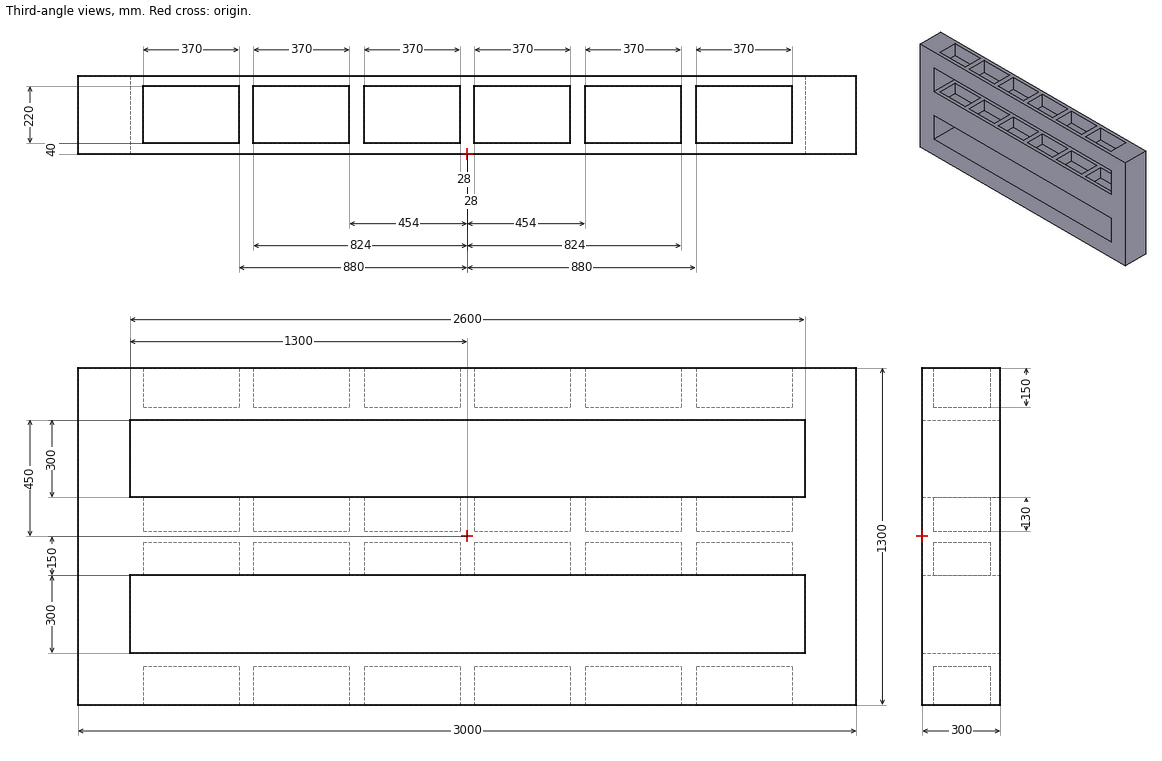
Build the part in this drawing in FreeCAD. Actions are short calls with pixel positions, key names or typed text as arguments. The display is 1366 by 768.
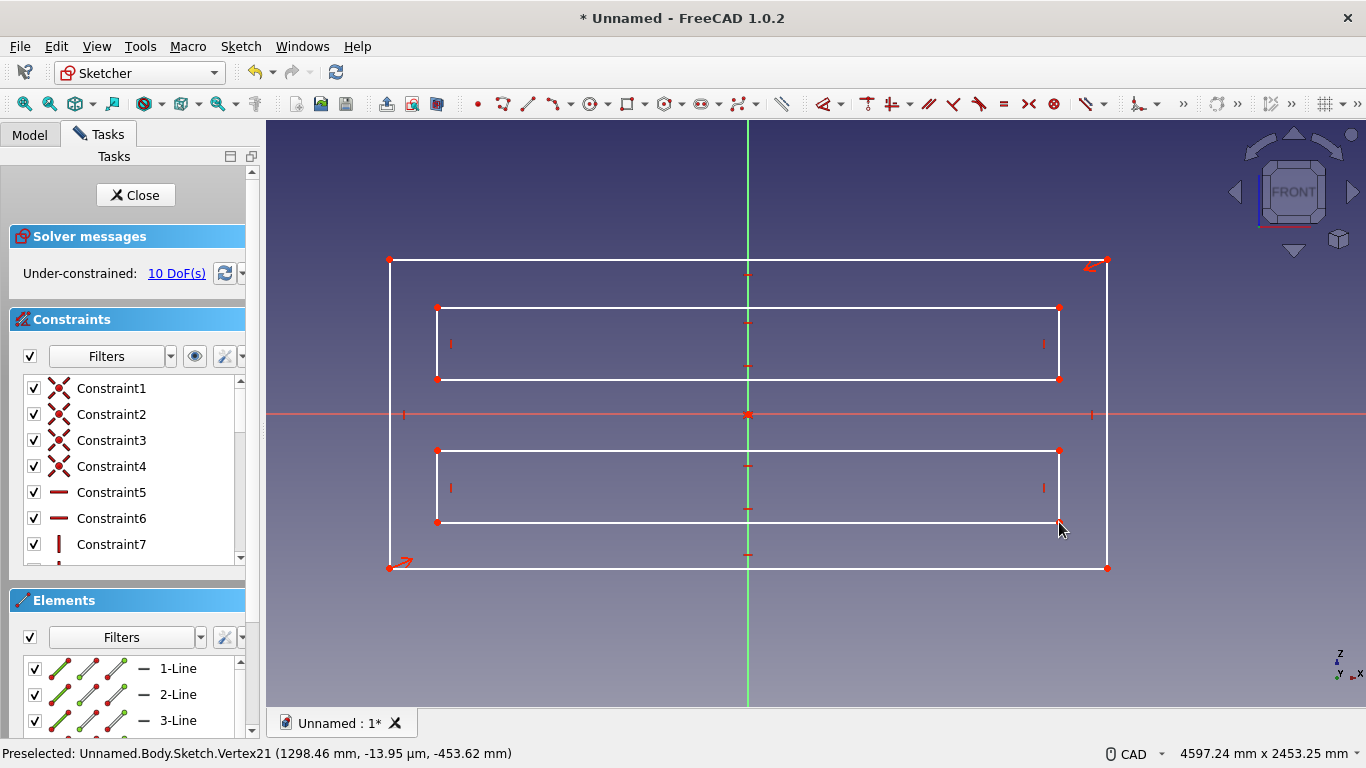
key(d)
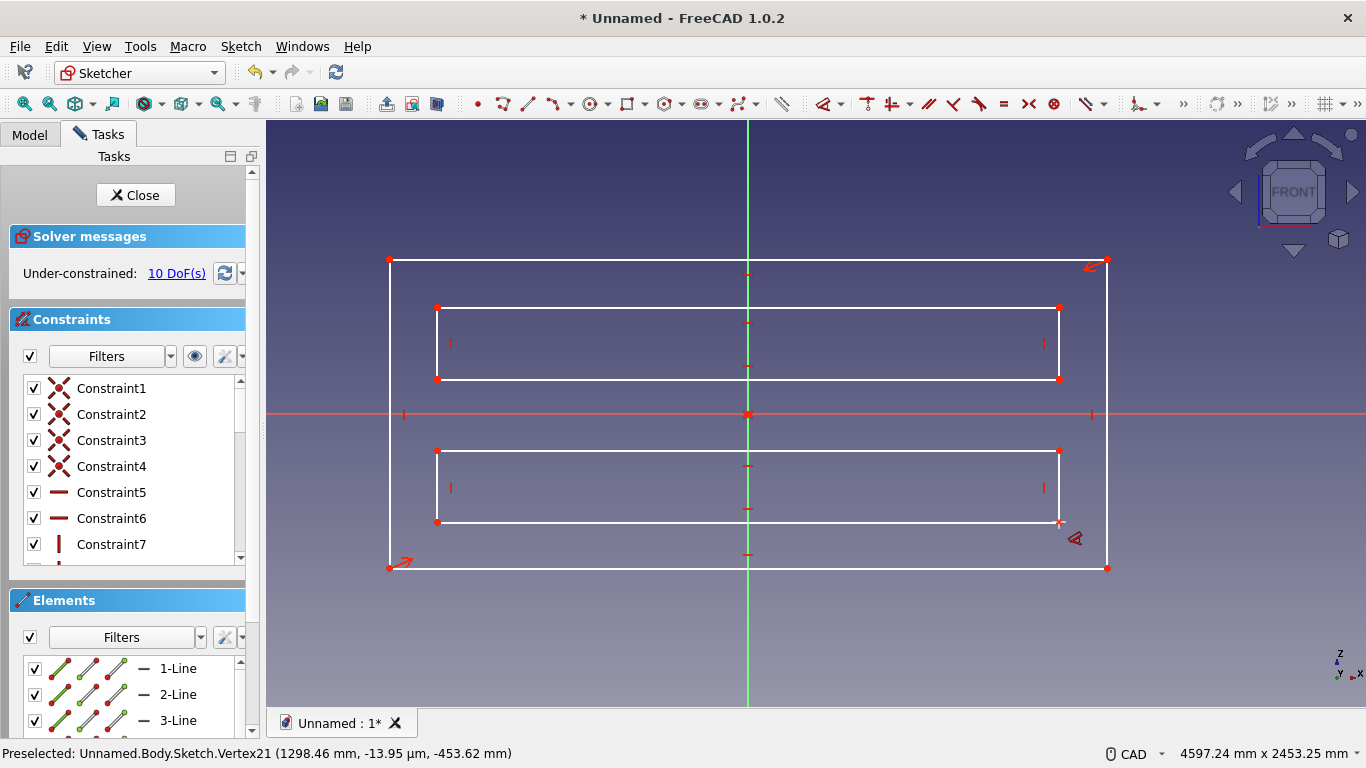
click(437, 330)
click(403, 344)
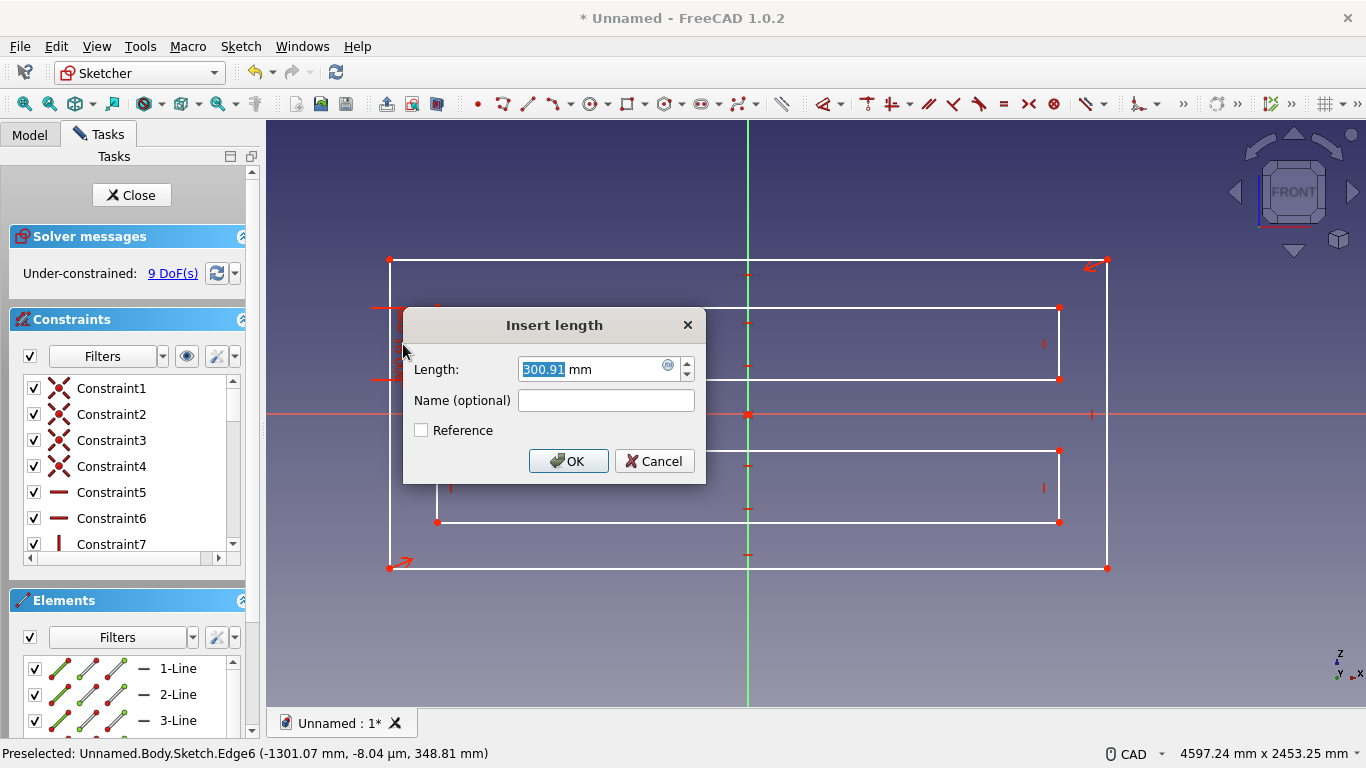
text(300)
key(Return)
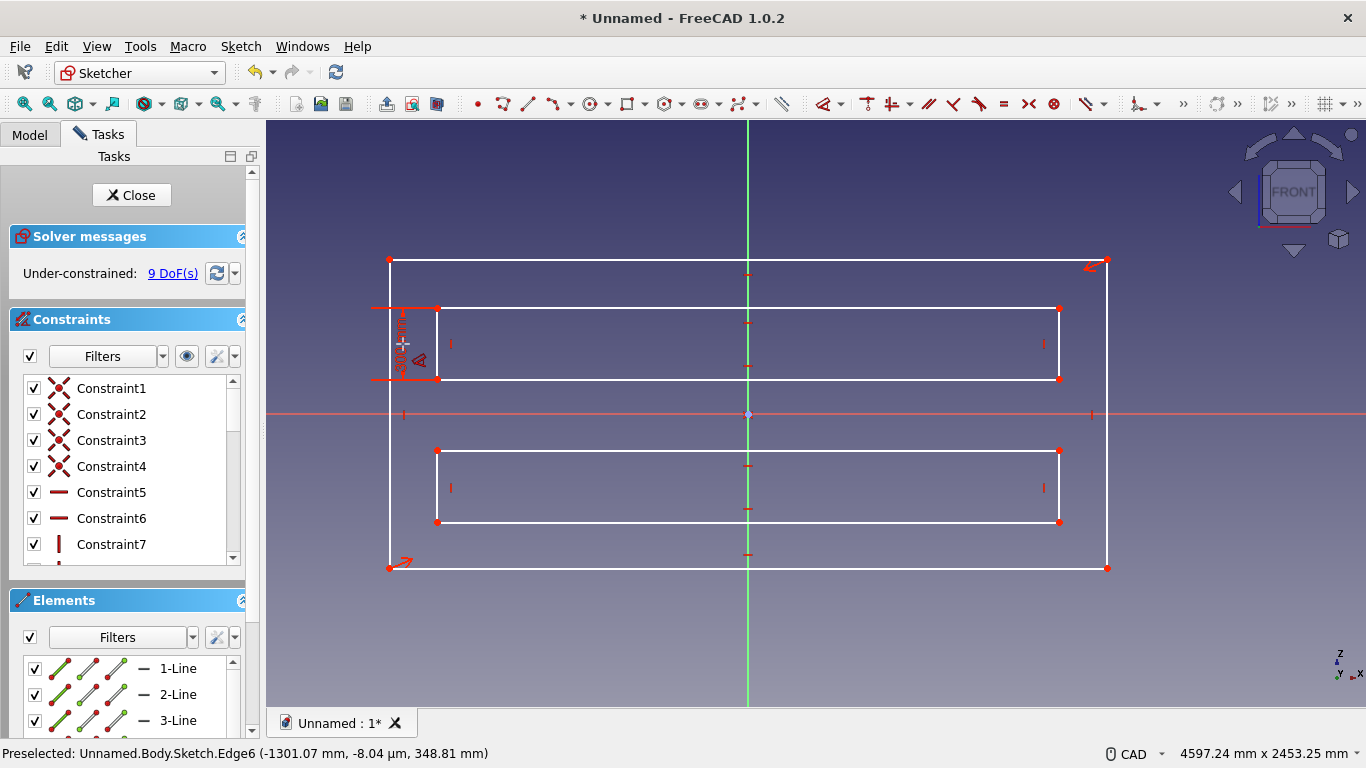
click(437, 473)
click(403, 487)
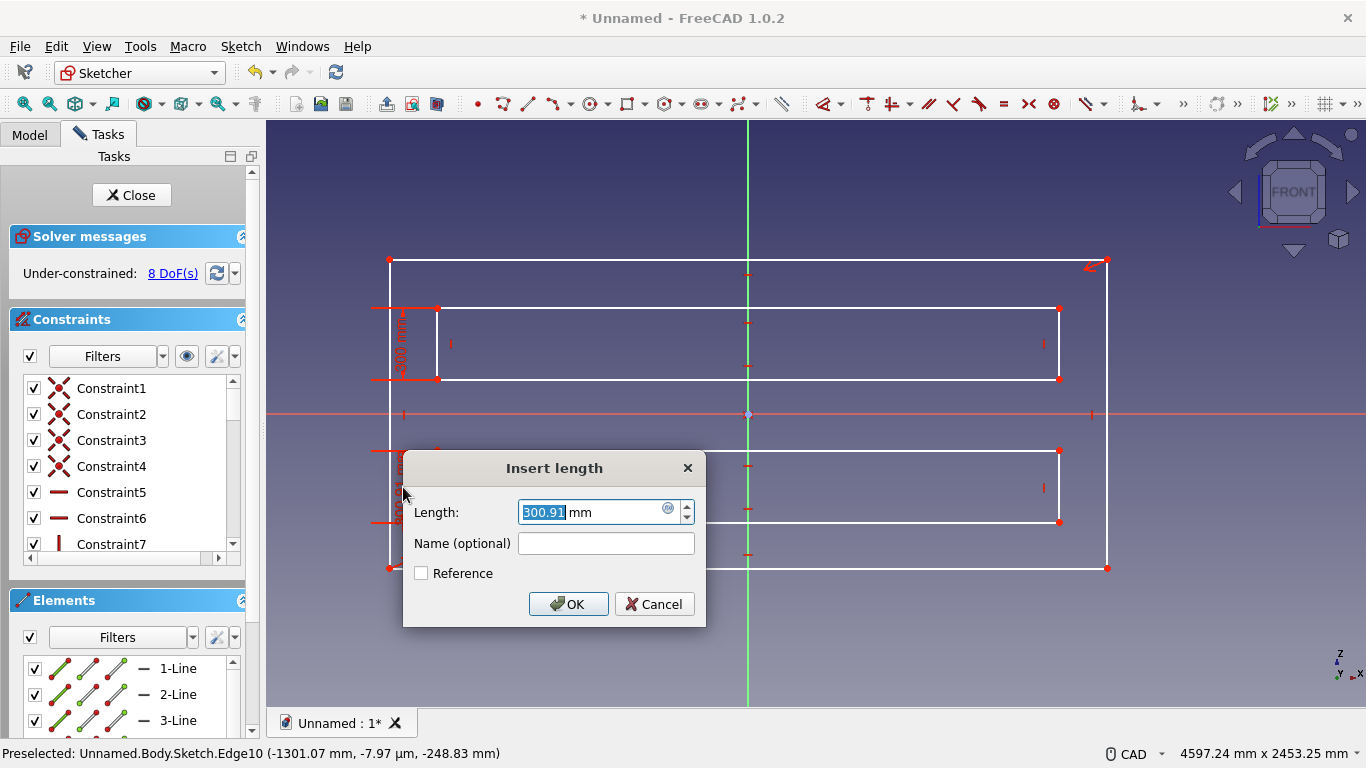
text(300)
key(Return)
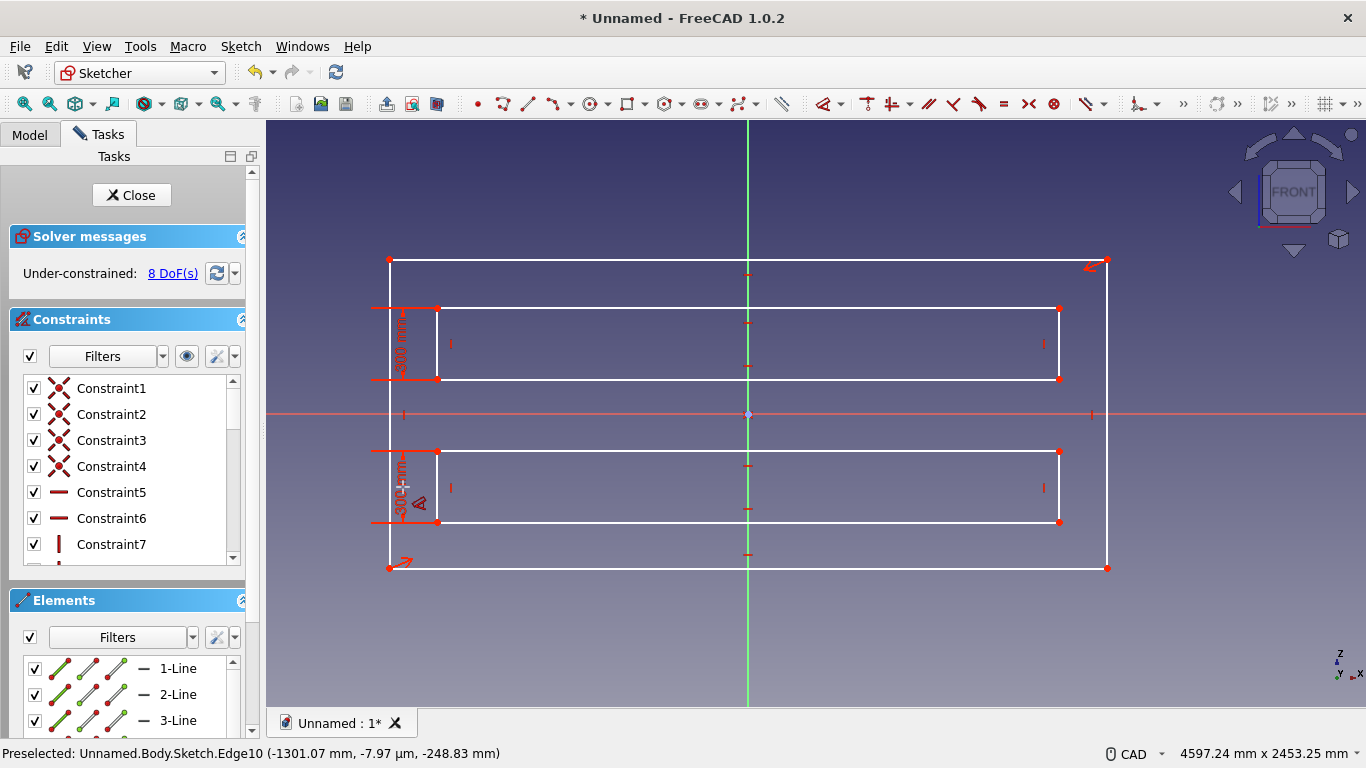
click(605, 569)
click(583, 603)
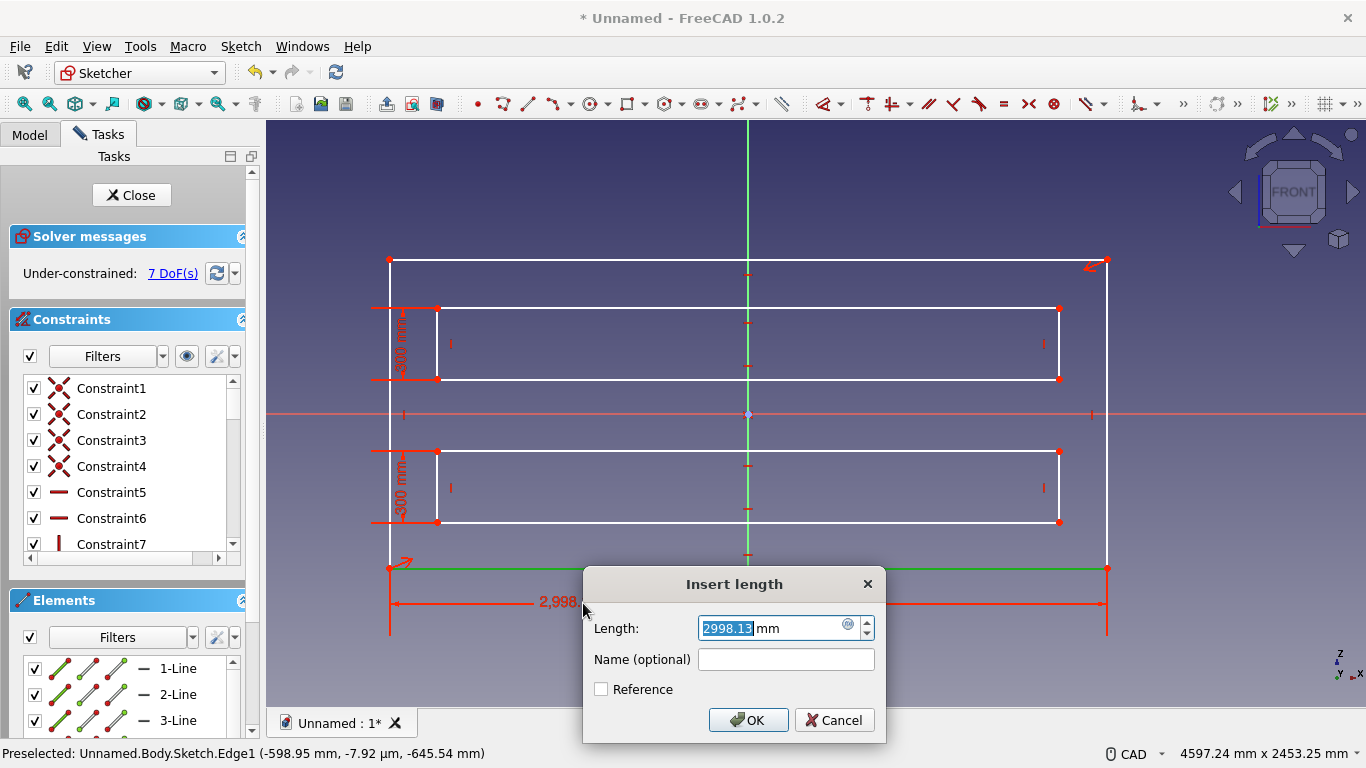
text(3000)
key(Return)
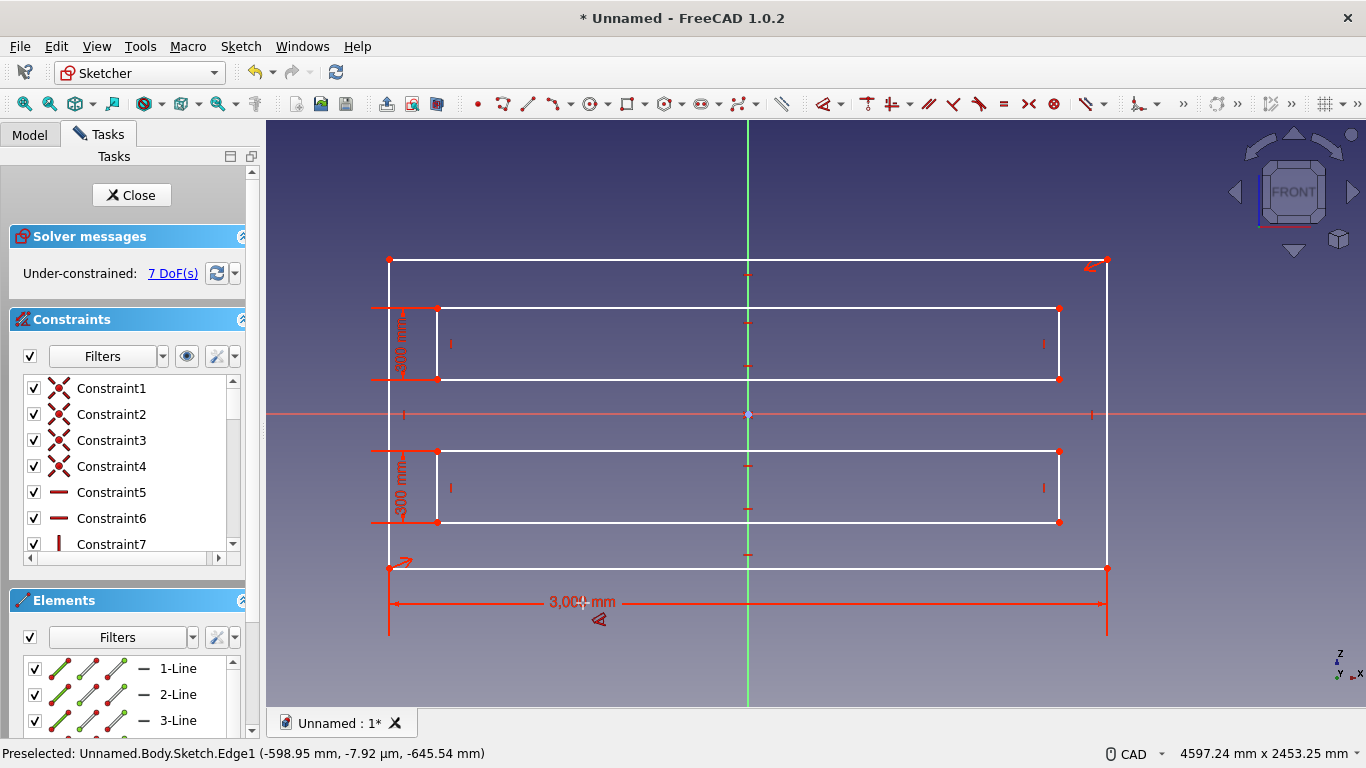
click(1107, 476)
click(1141, 343)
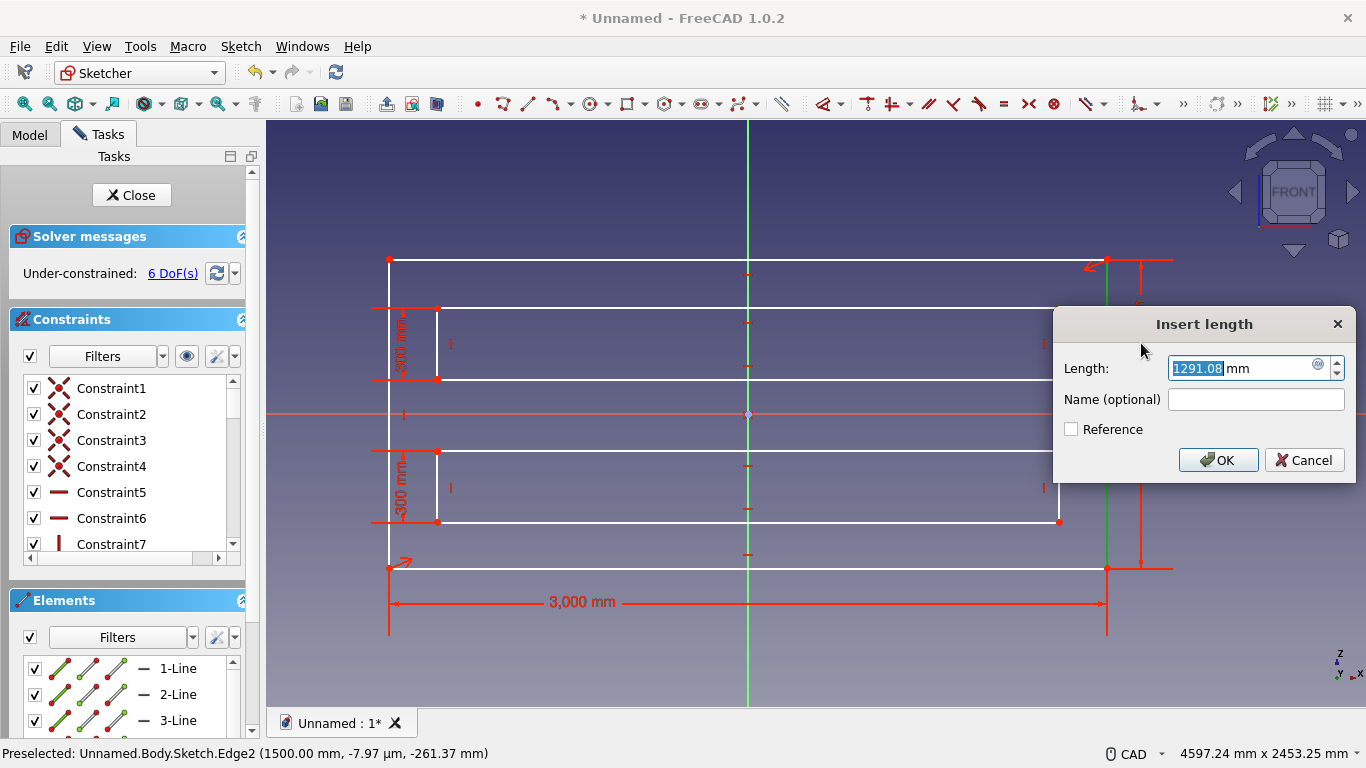
text(1300)
key(Return)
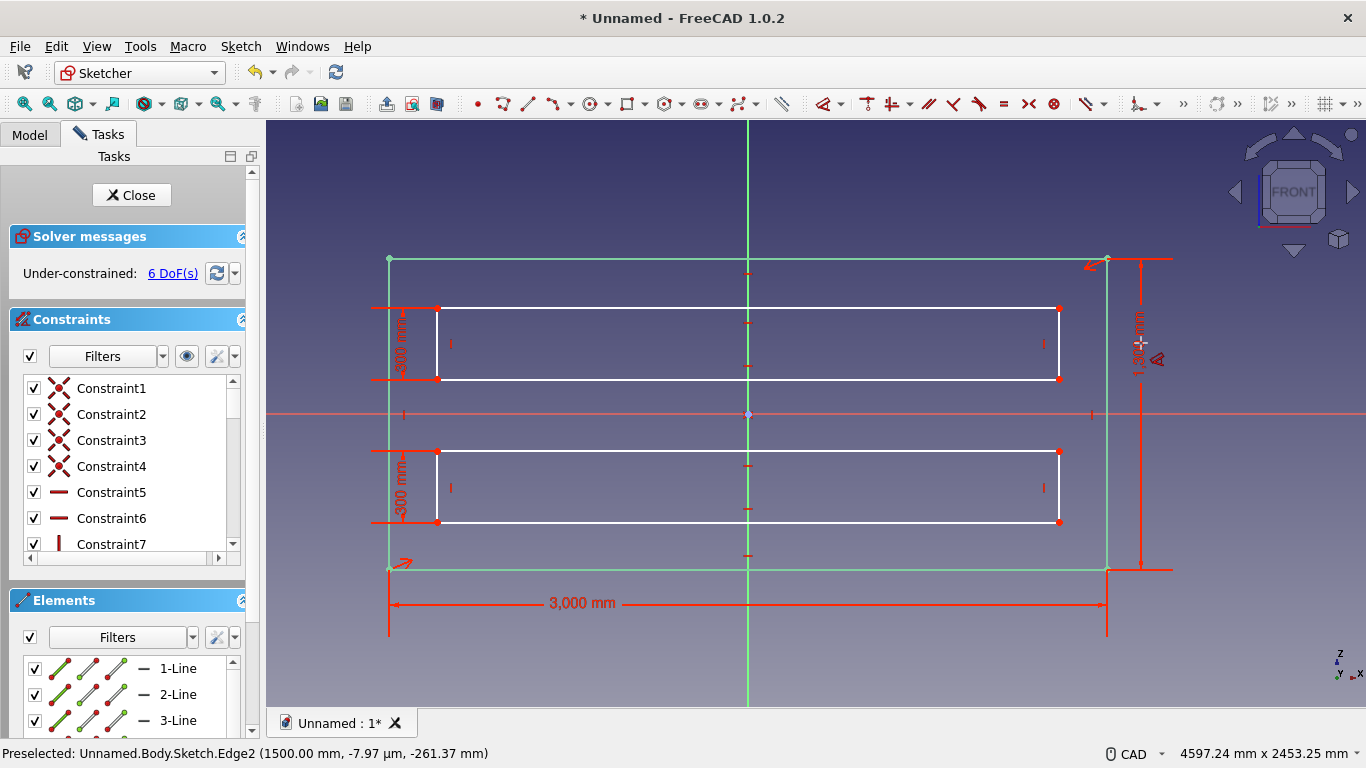
click(624, 380)
click(605, 346)